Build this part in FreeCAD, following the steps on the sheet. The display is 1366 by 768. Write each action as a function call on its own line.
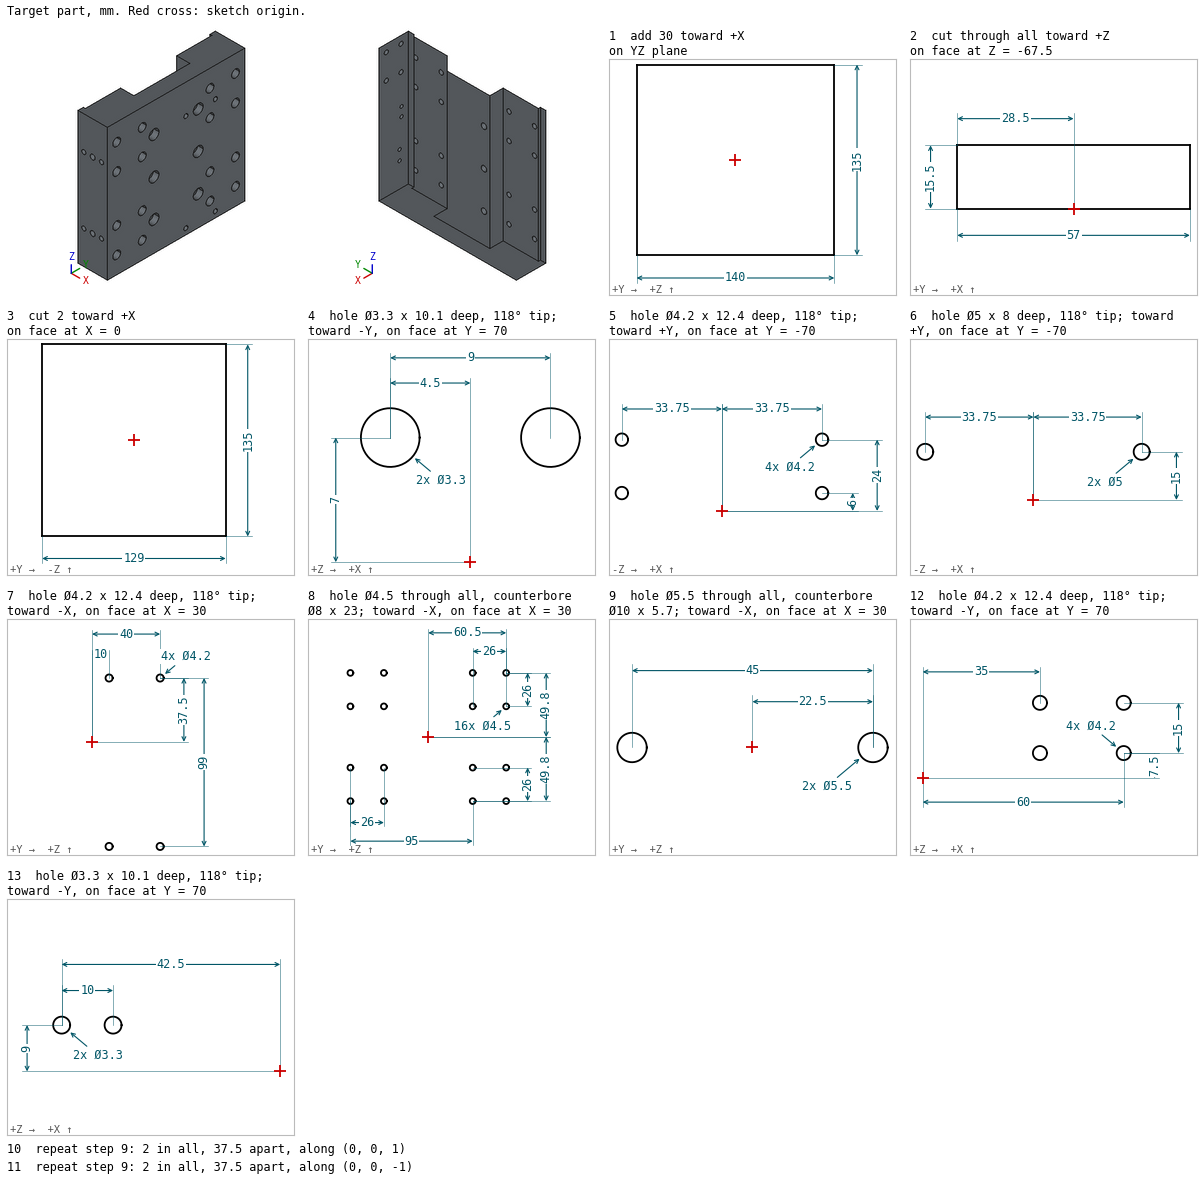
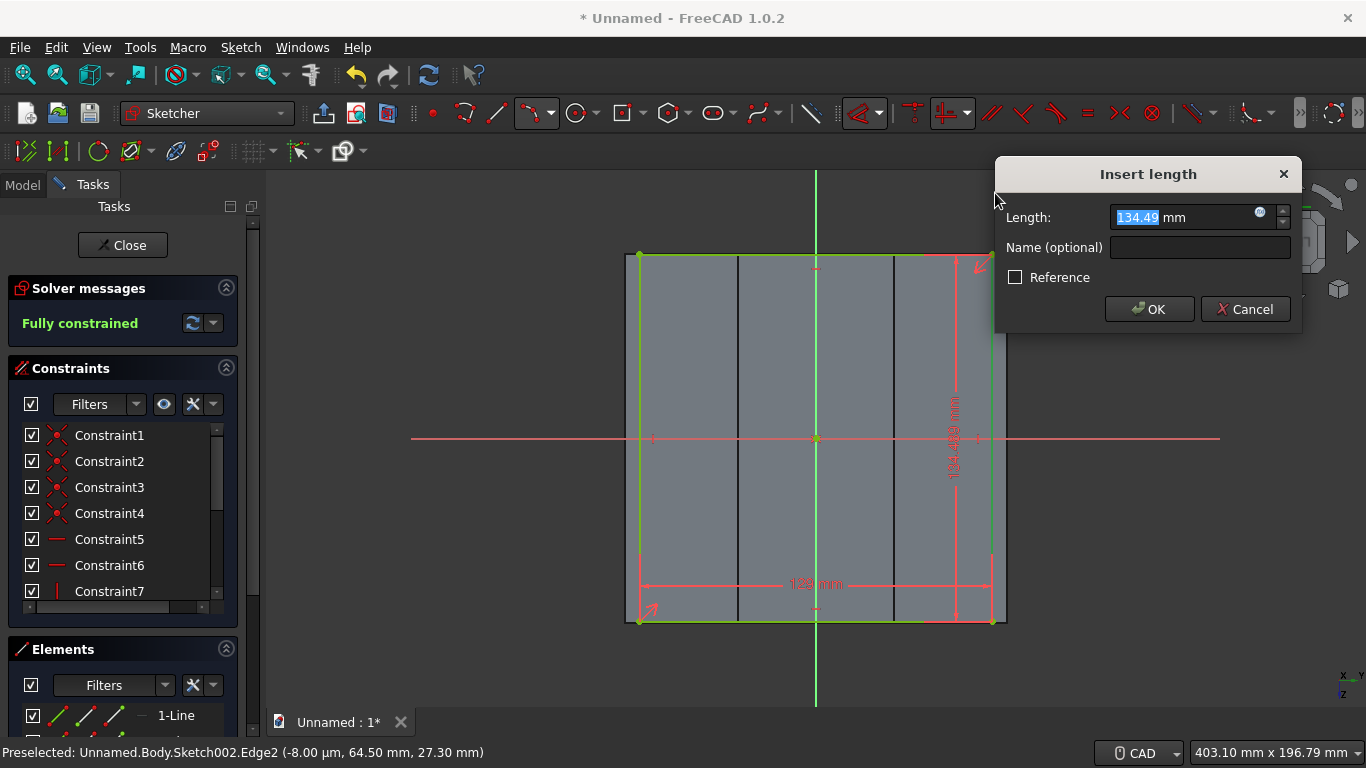
text(135)
key(Return)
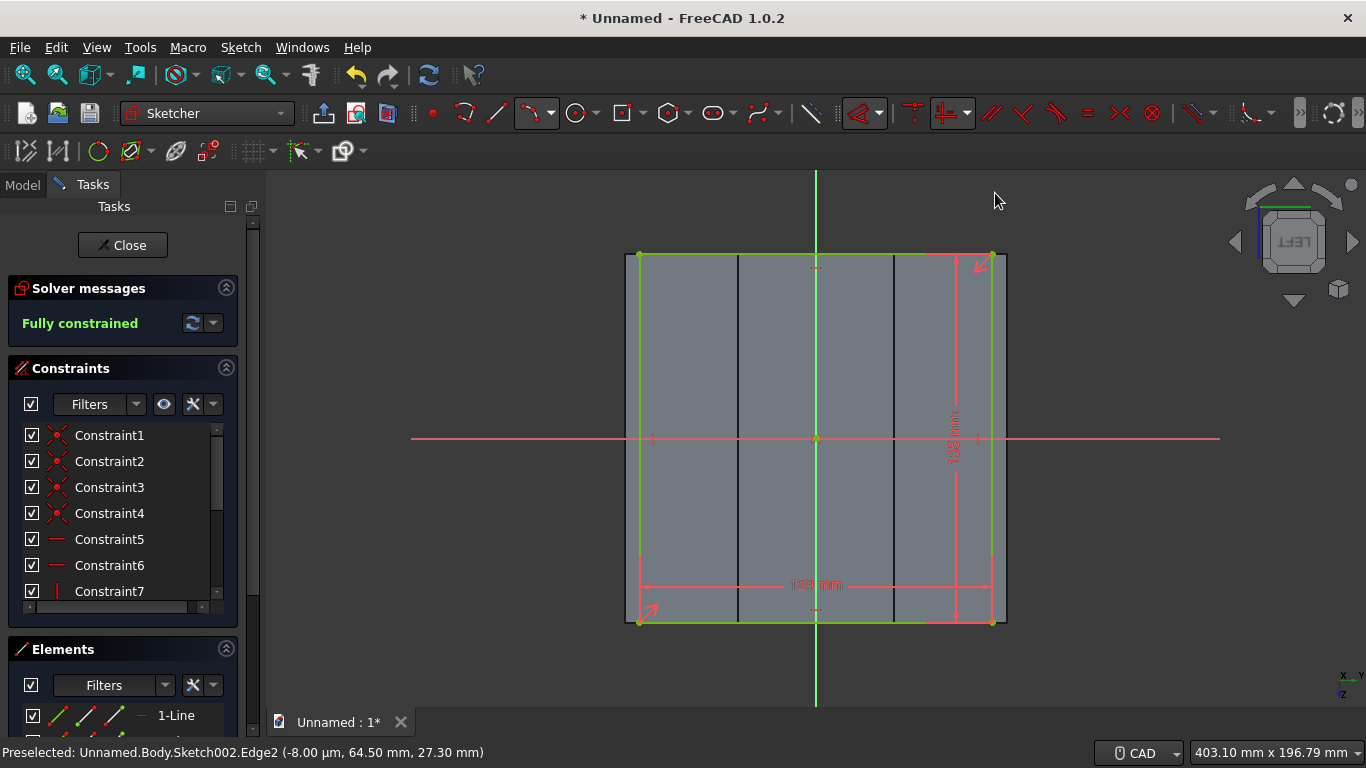
click(123, 245)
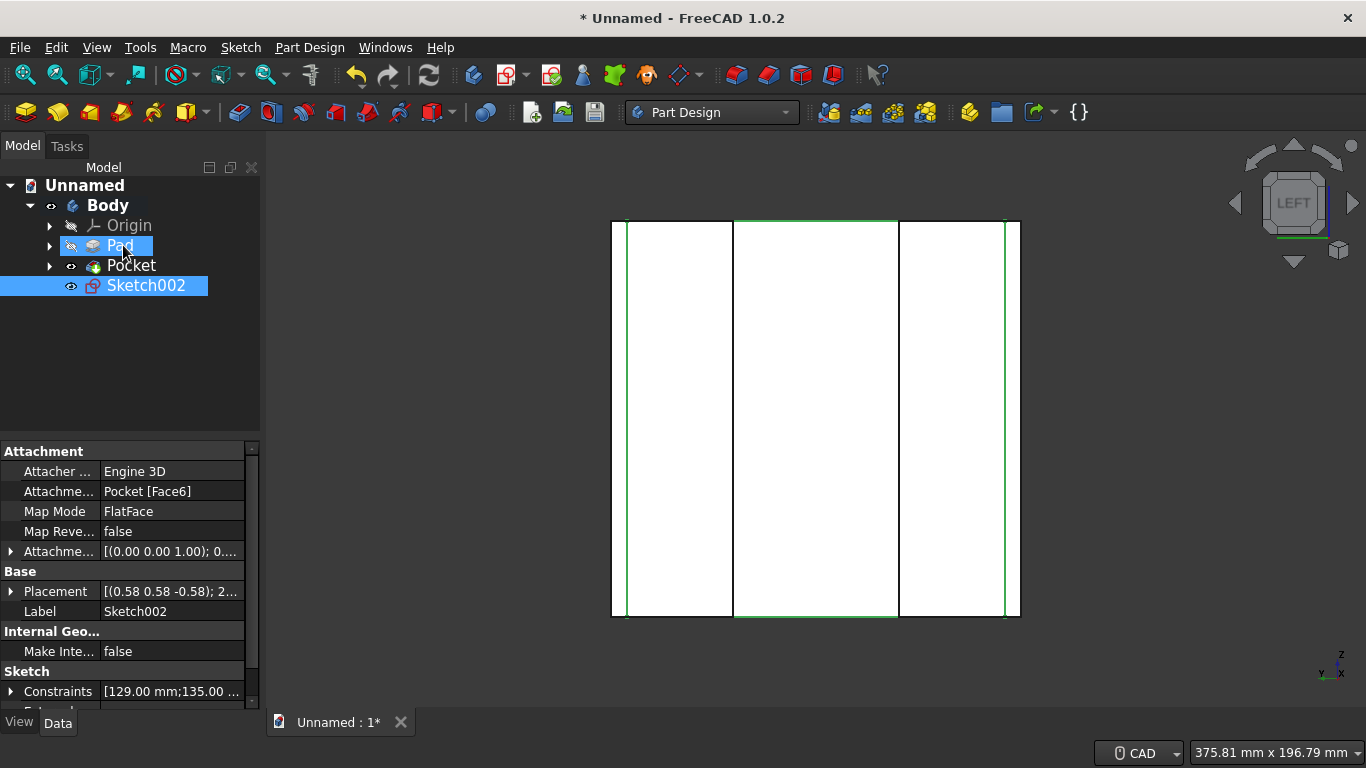
click(240, 112)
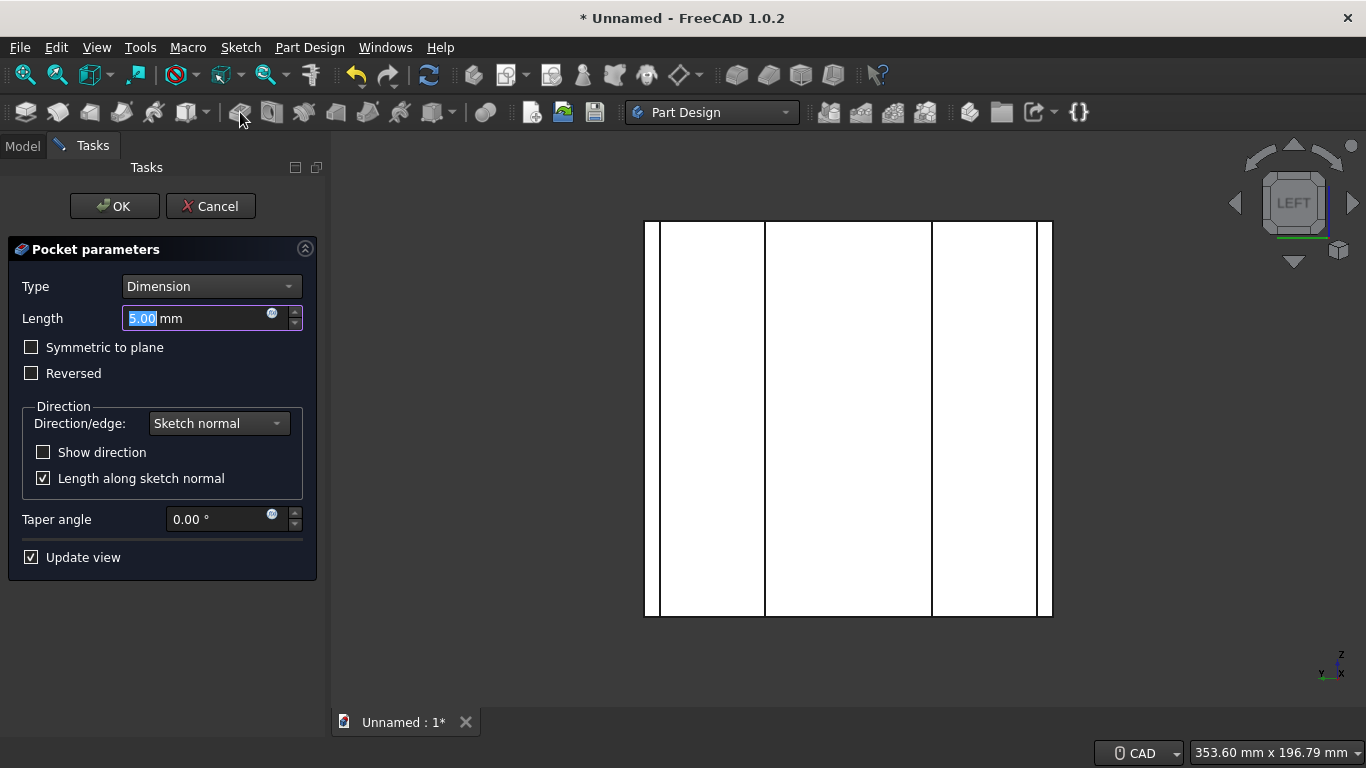
text(2)
key(Tab)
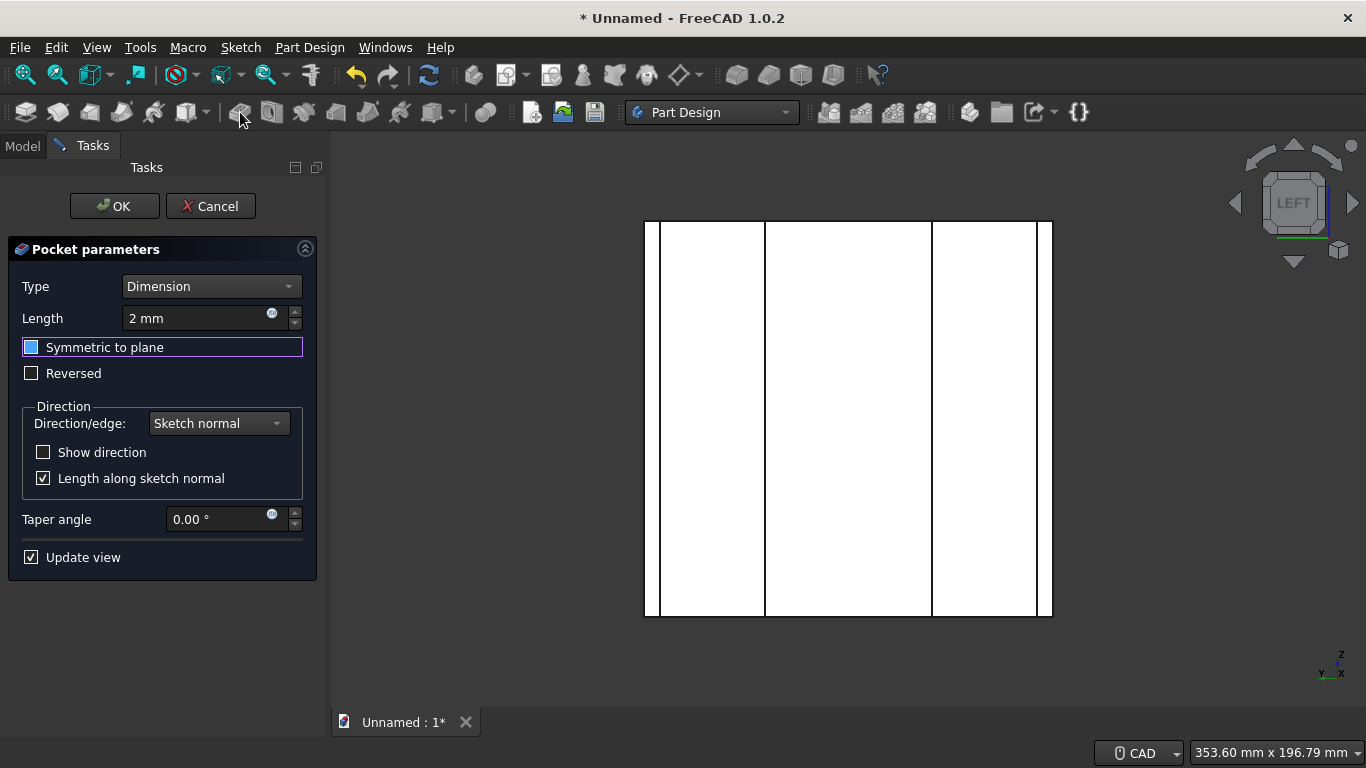
click(115, 206)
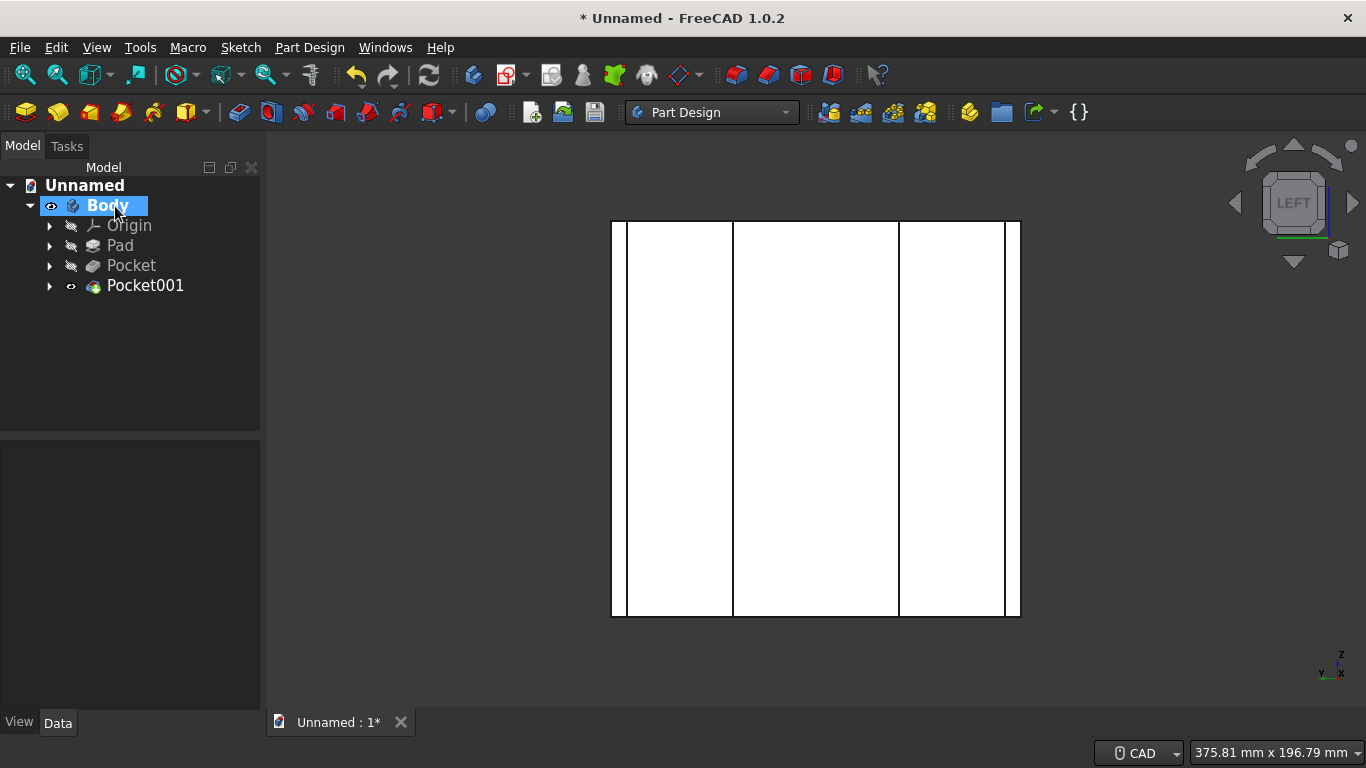
key(4)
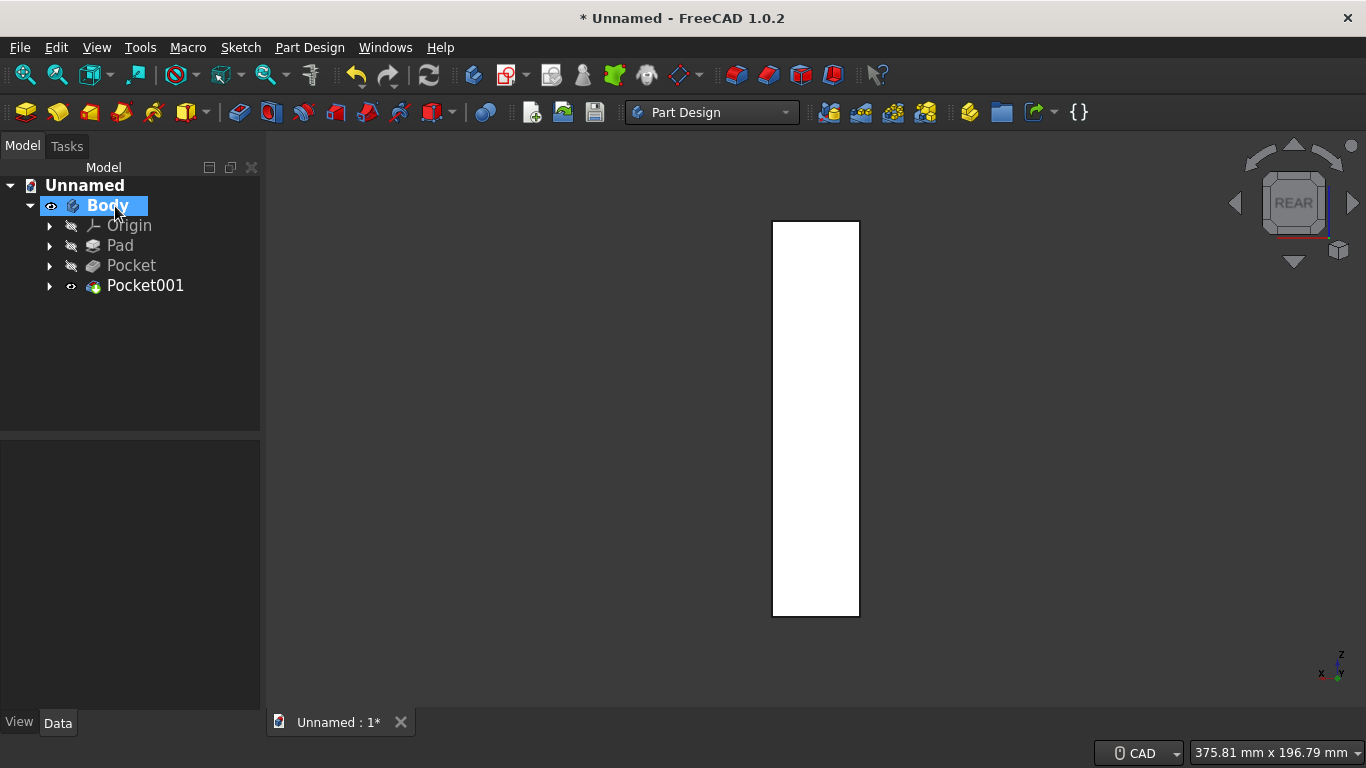
click(816, 418)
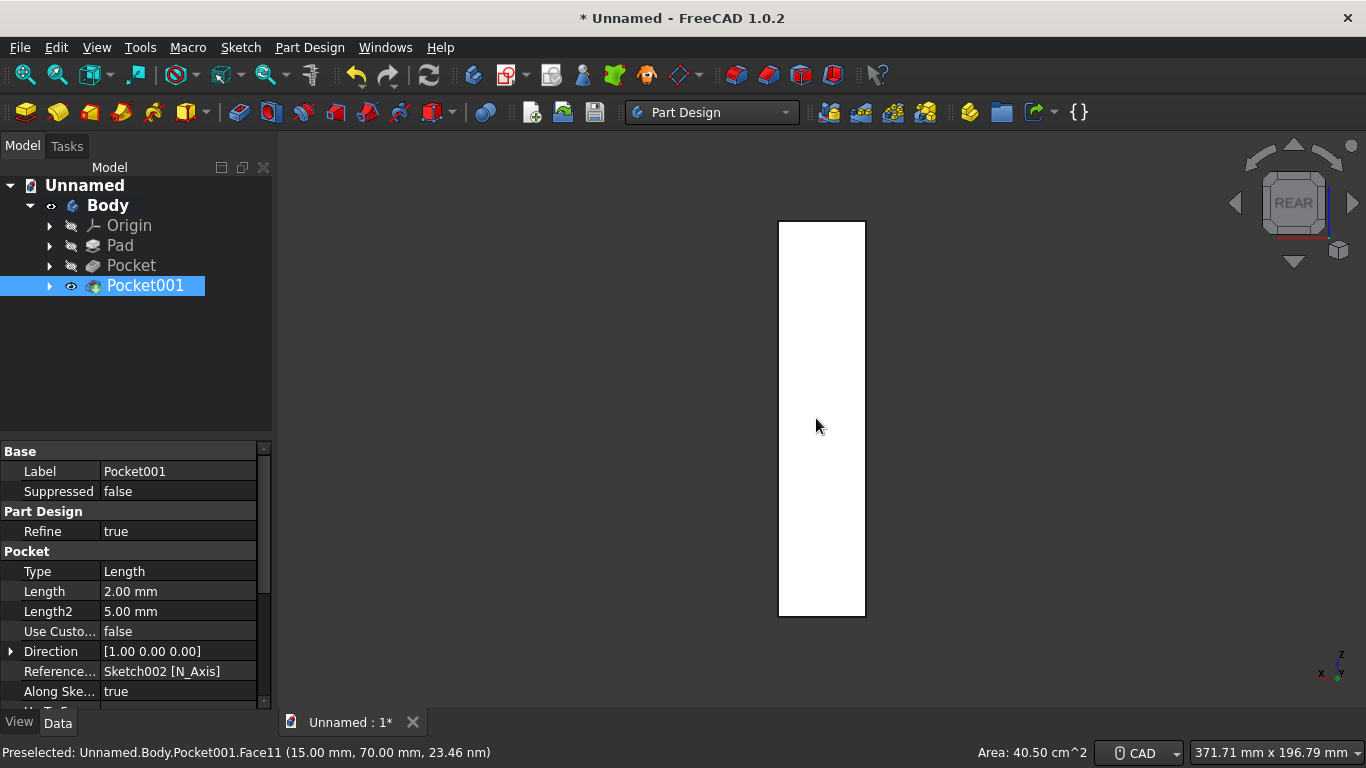
click(506, 76)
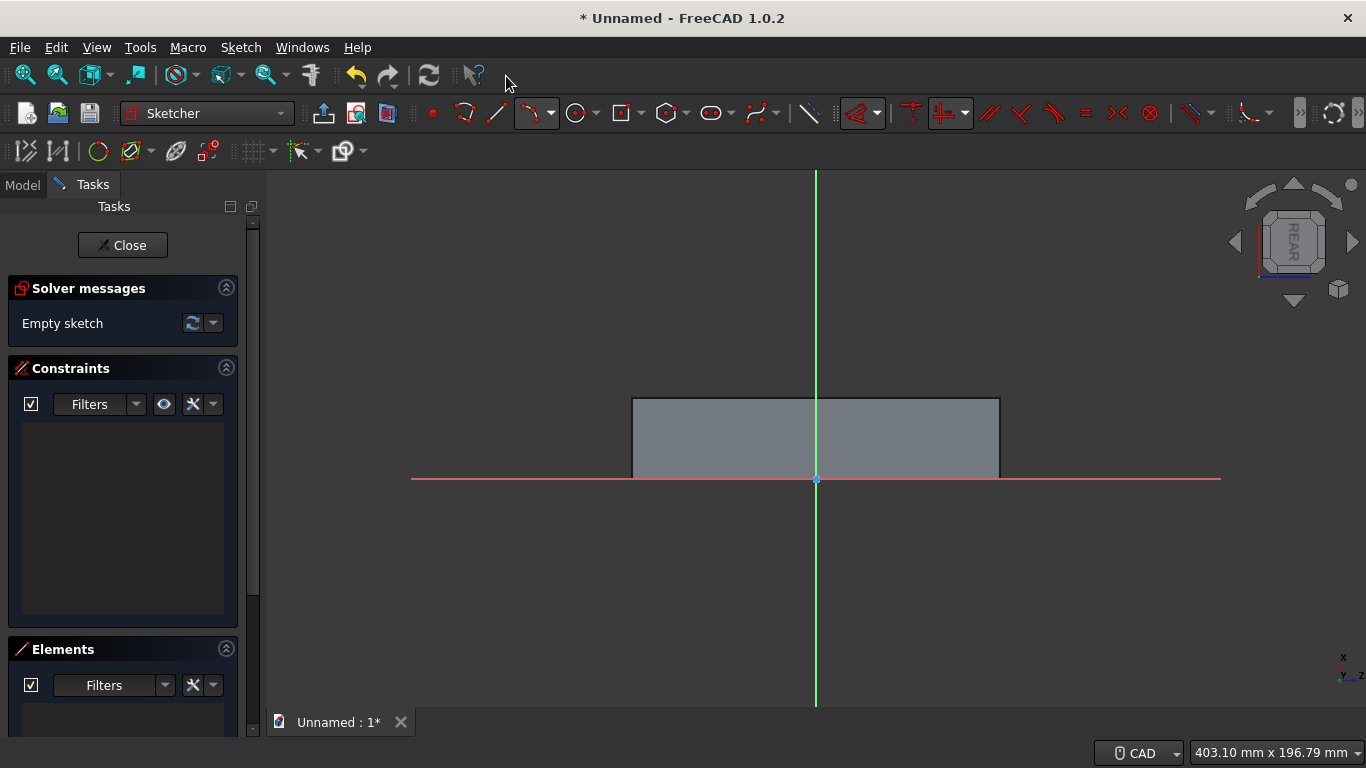
scroll(821, 470, up, 13)